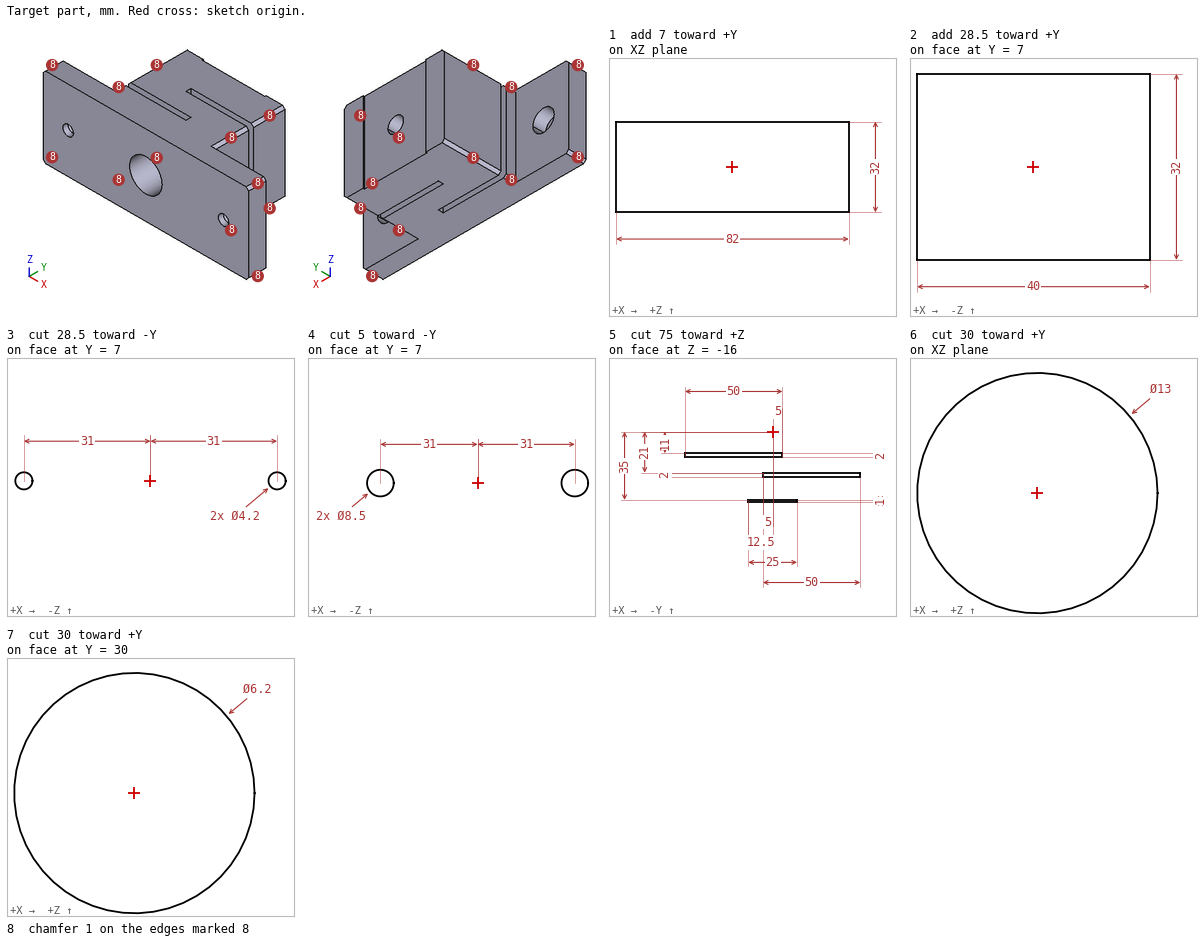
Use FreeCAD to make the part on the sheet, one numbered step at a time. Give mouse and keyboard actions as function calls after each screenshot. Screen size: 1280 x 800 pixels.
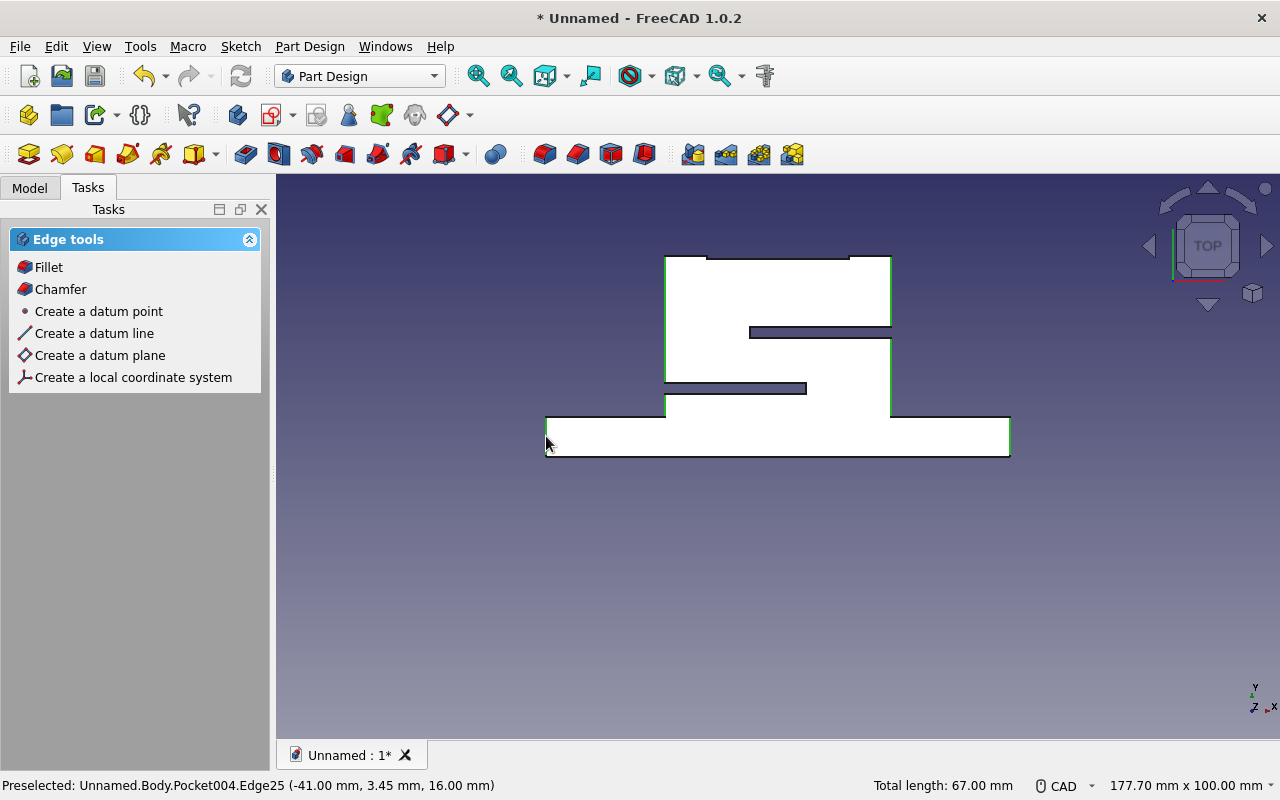
key(1)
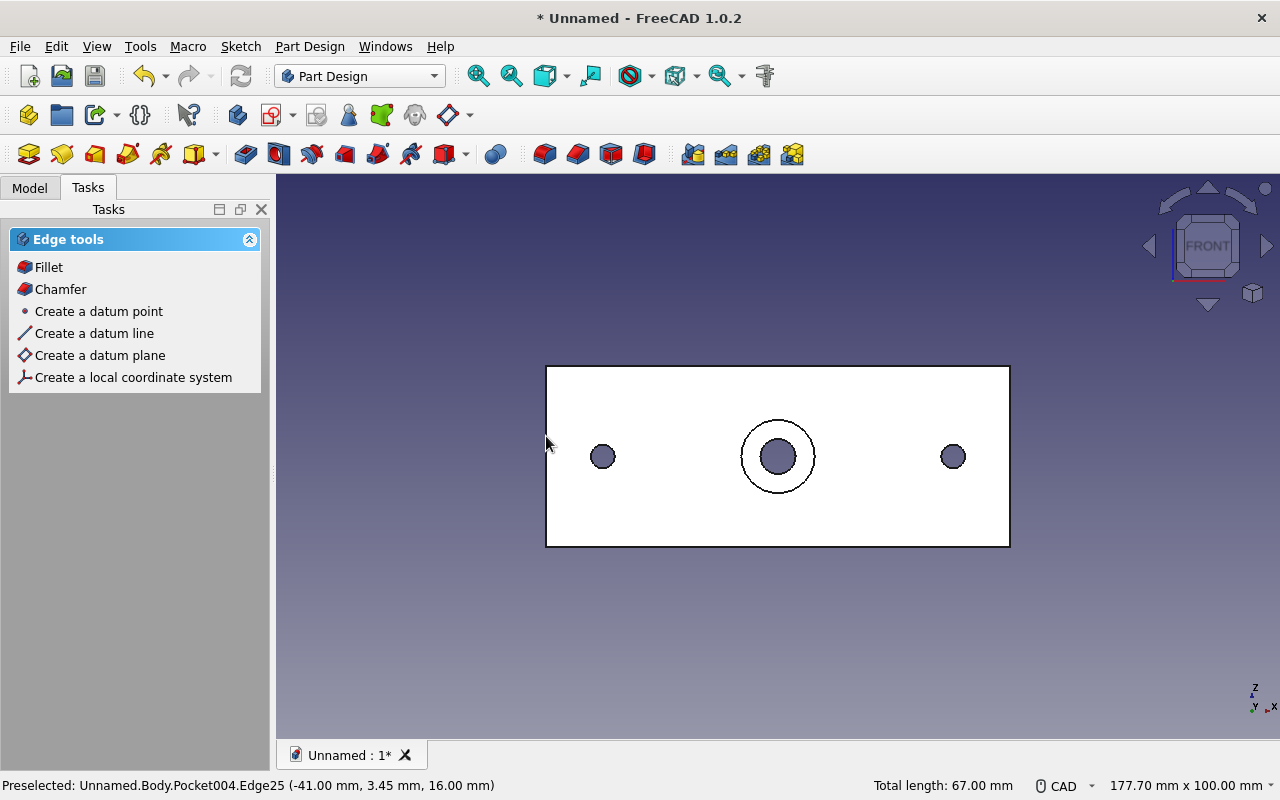
key(3)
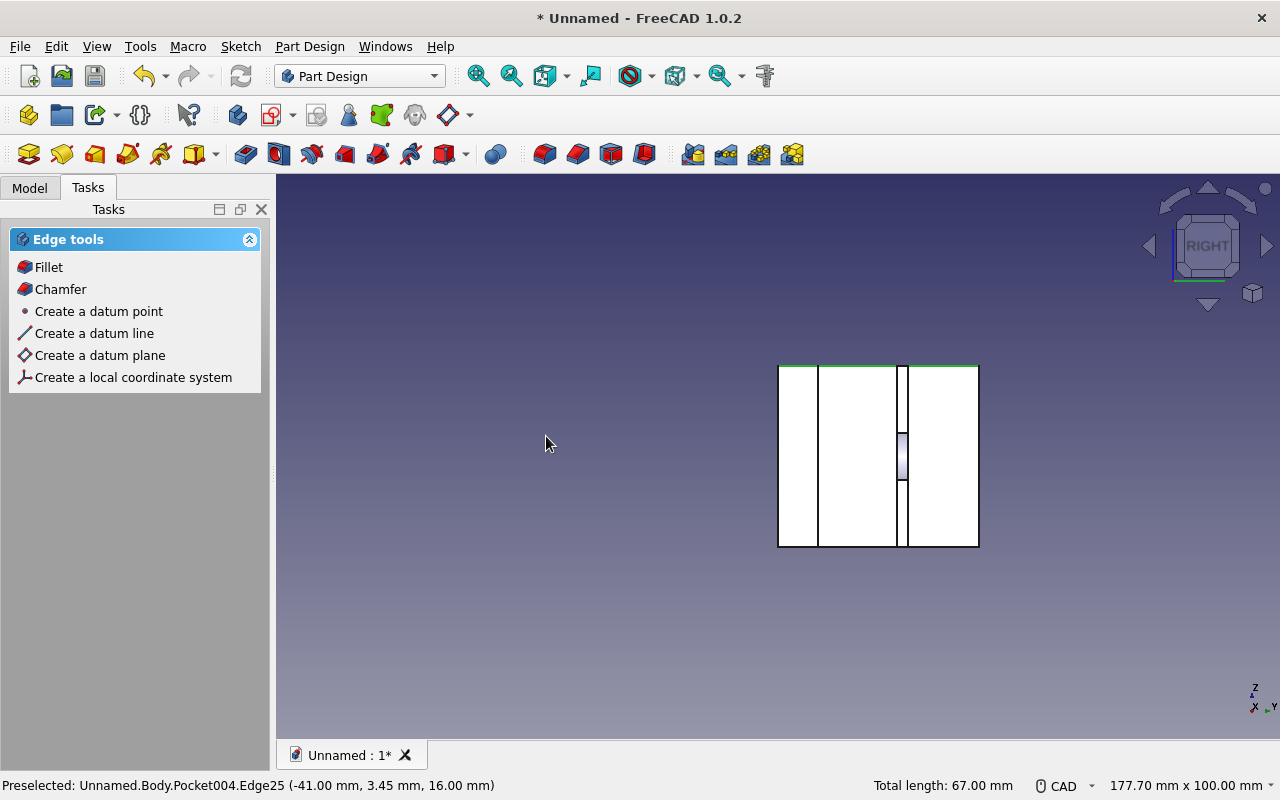
key(v)
key(f)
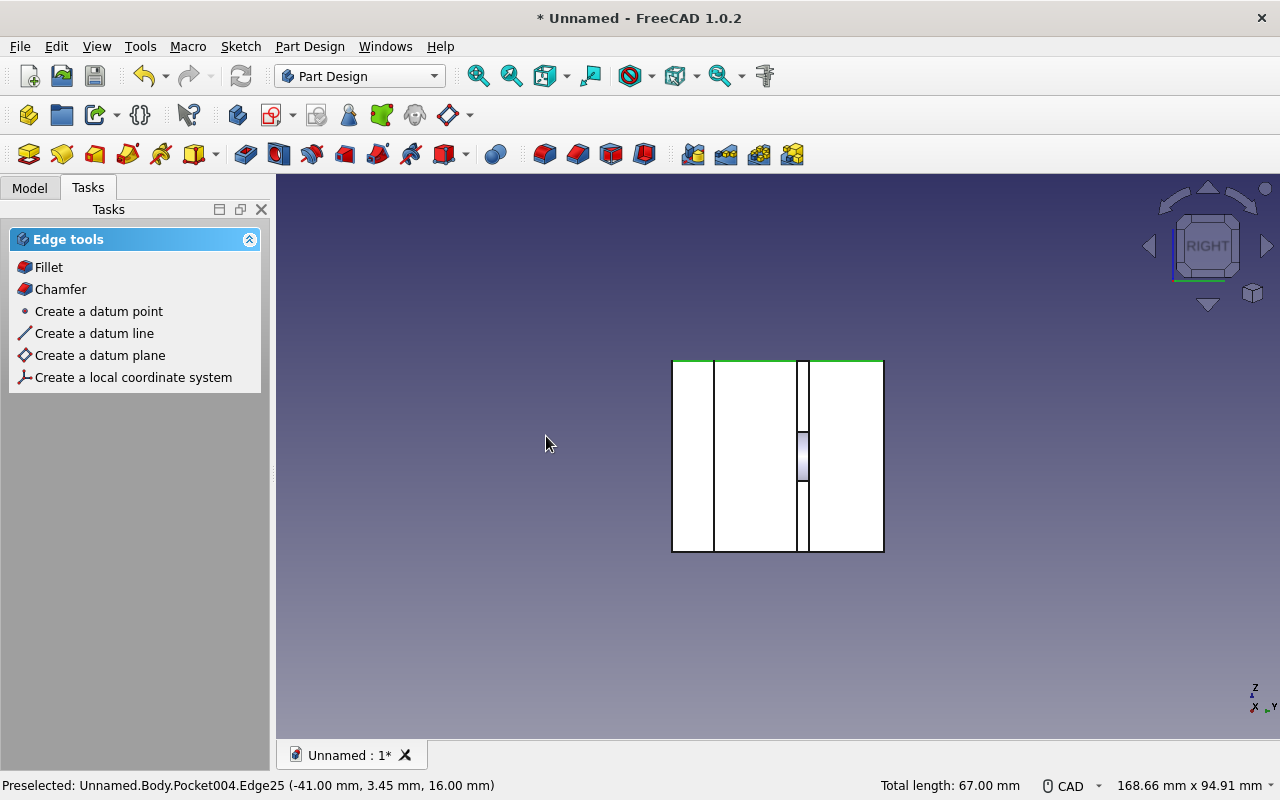
click(846, 551, ctrl)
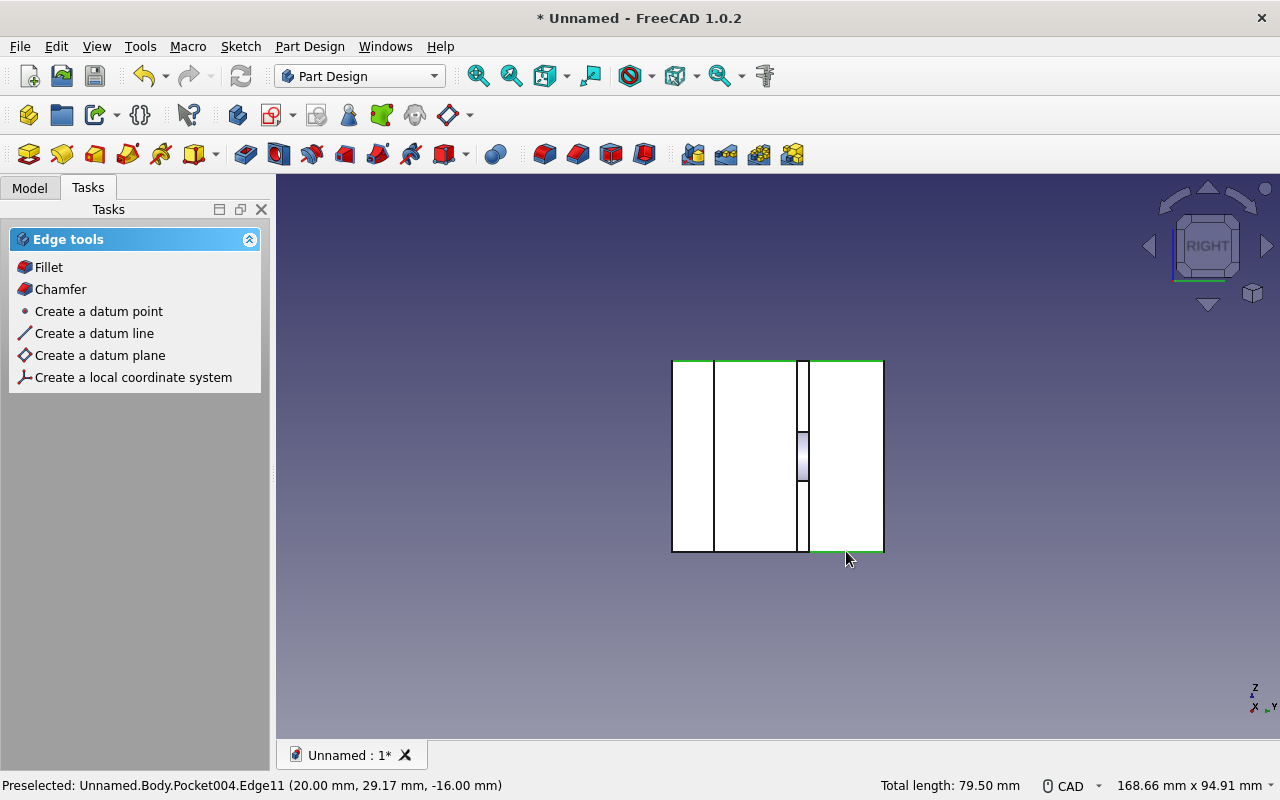
click(756, 551, ctrl)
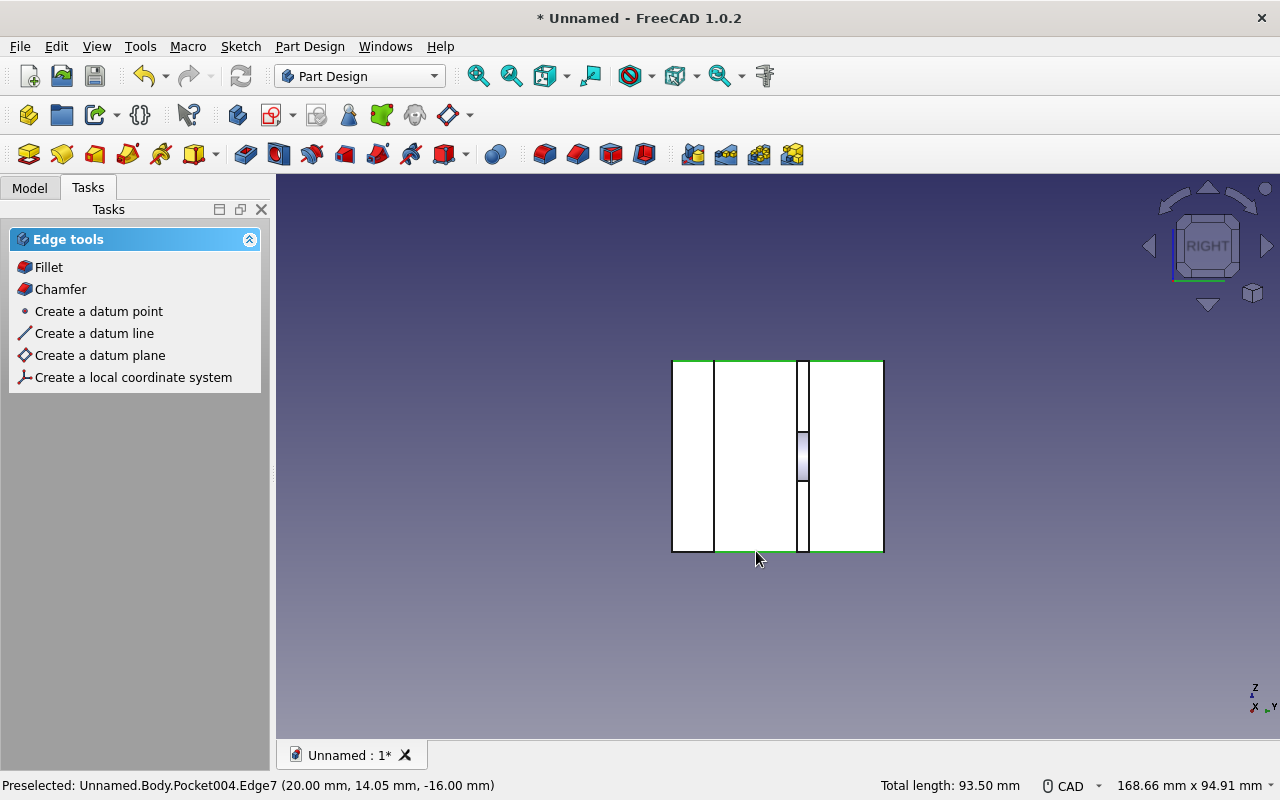
click(693, 551, ctrl)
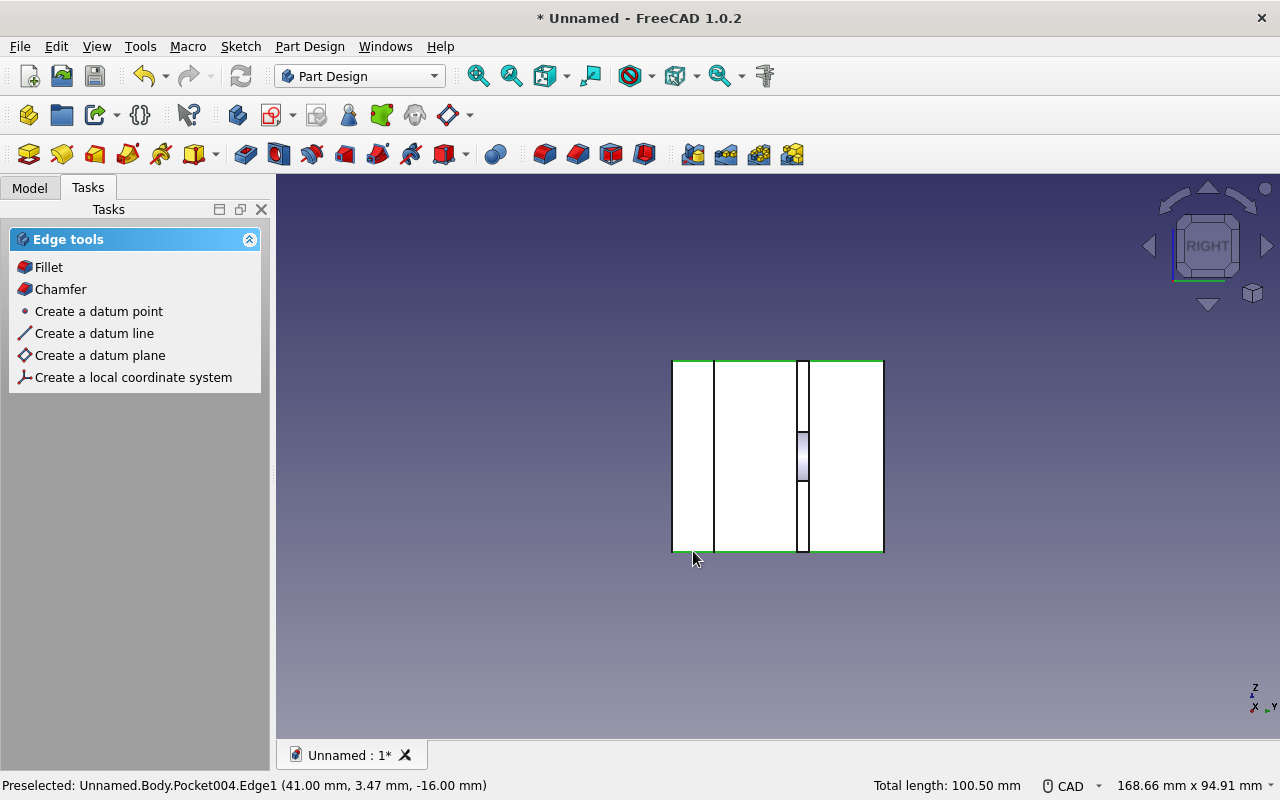
key(5)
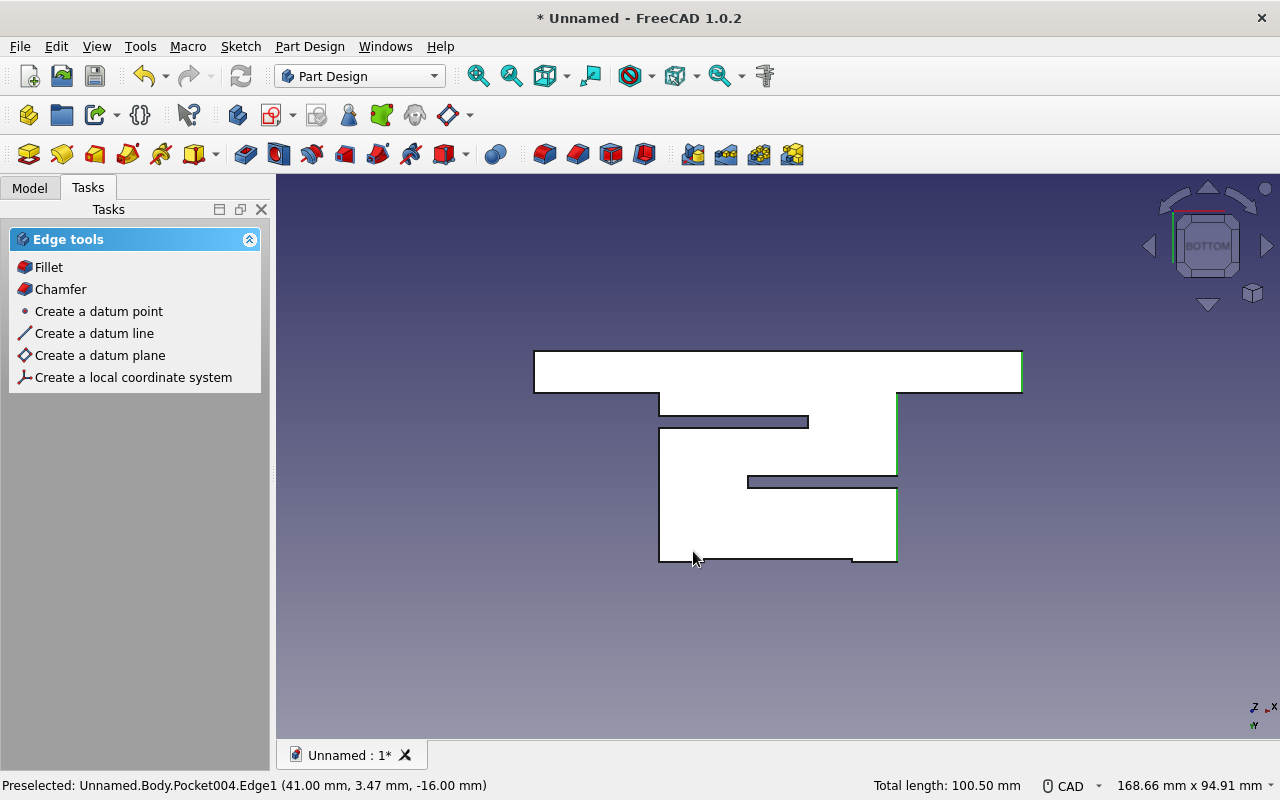
click(659, 494, ctrl)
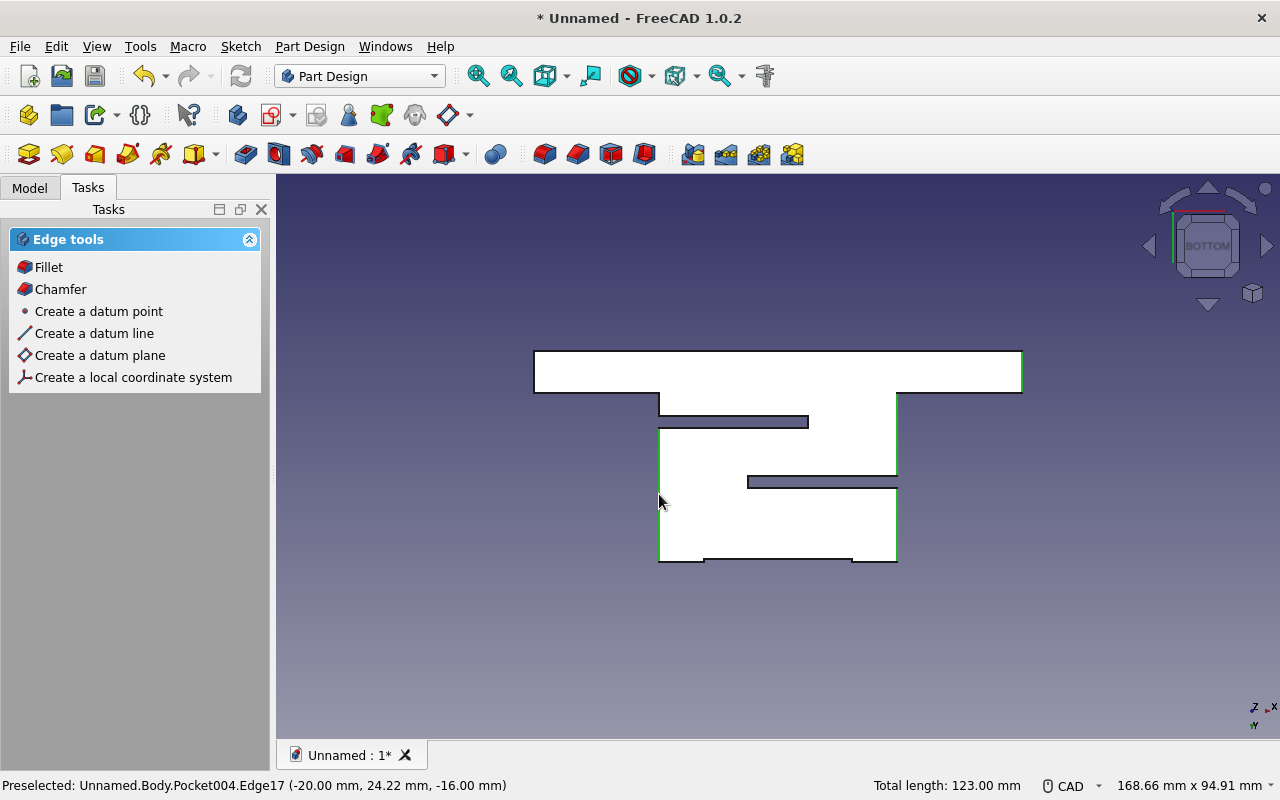
click(659, 403, ctrl)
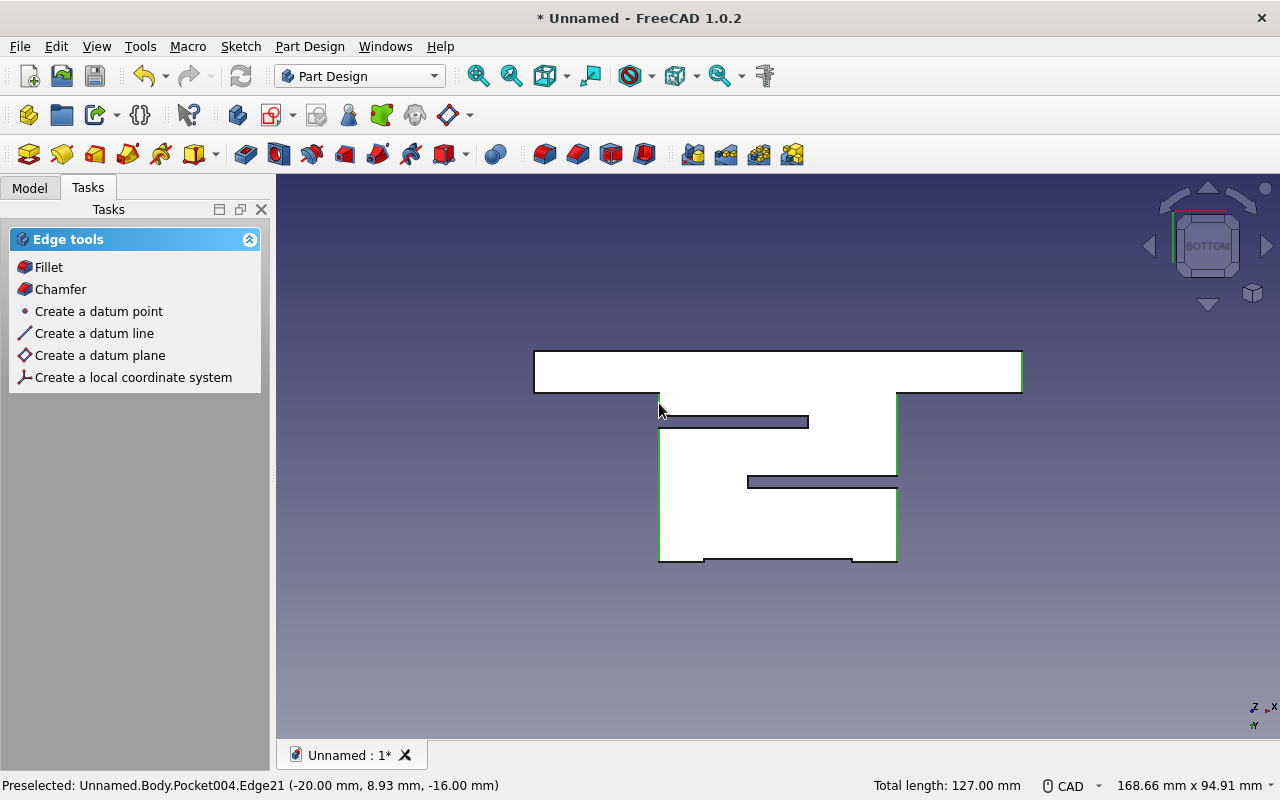
click(534, 371, ctrl)